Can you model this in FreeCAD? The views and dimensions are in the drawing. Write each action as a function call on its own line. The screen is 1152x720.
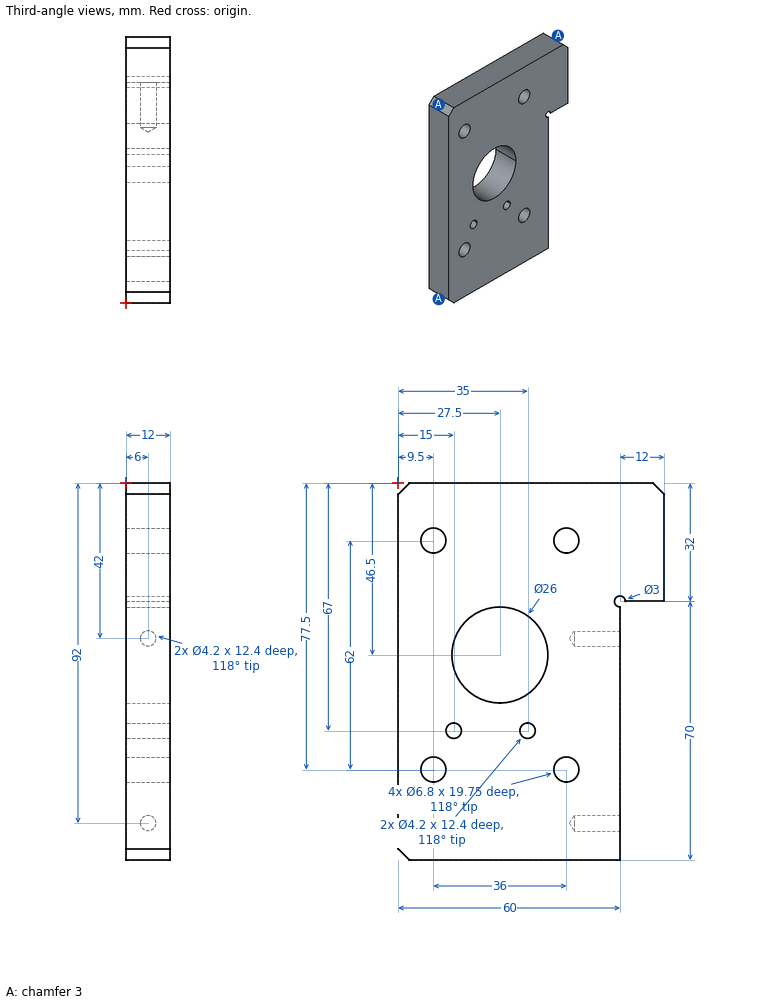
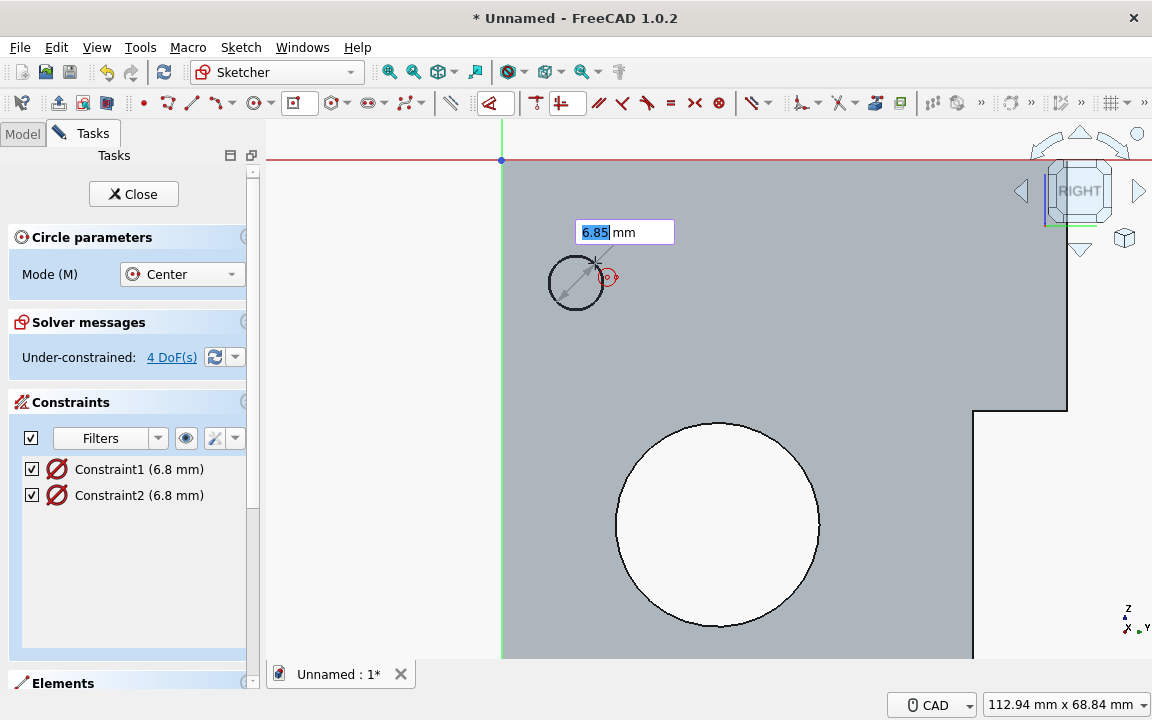
text(6.8)
key(Return)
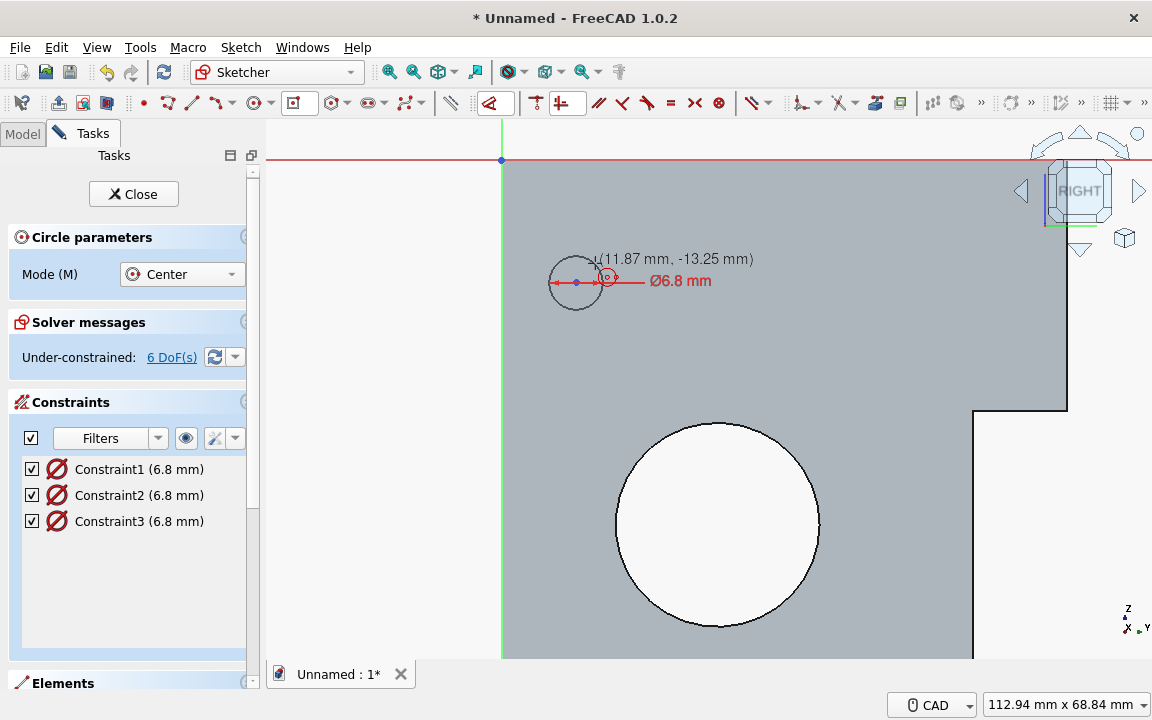
click(859, 282)
move(878, 263)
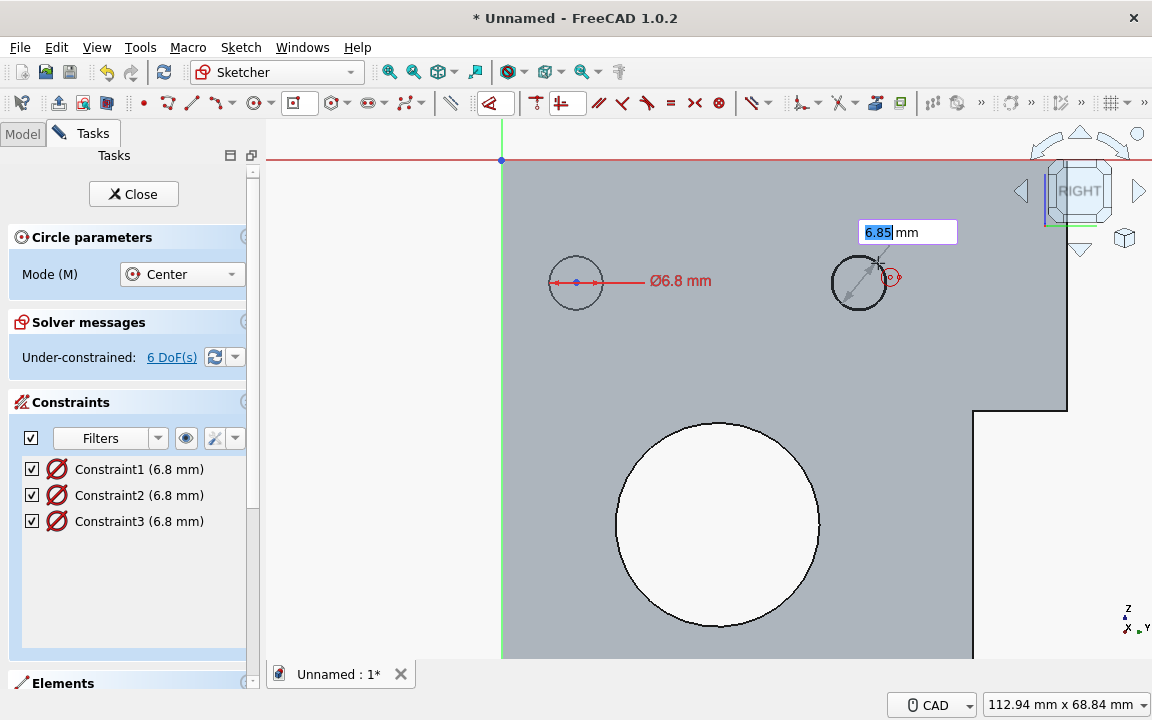
text(6.8)
key(Return)
key(Escape)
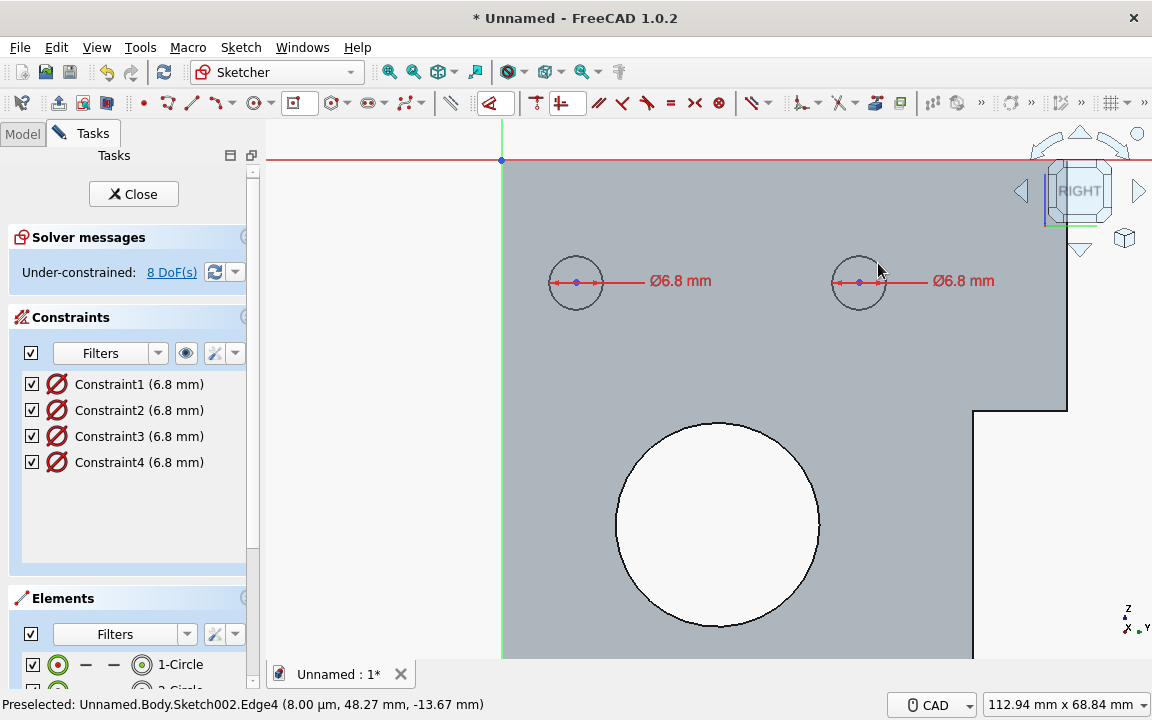
scroll(576, 281, down, 3)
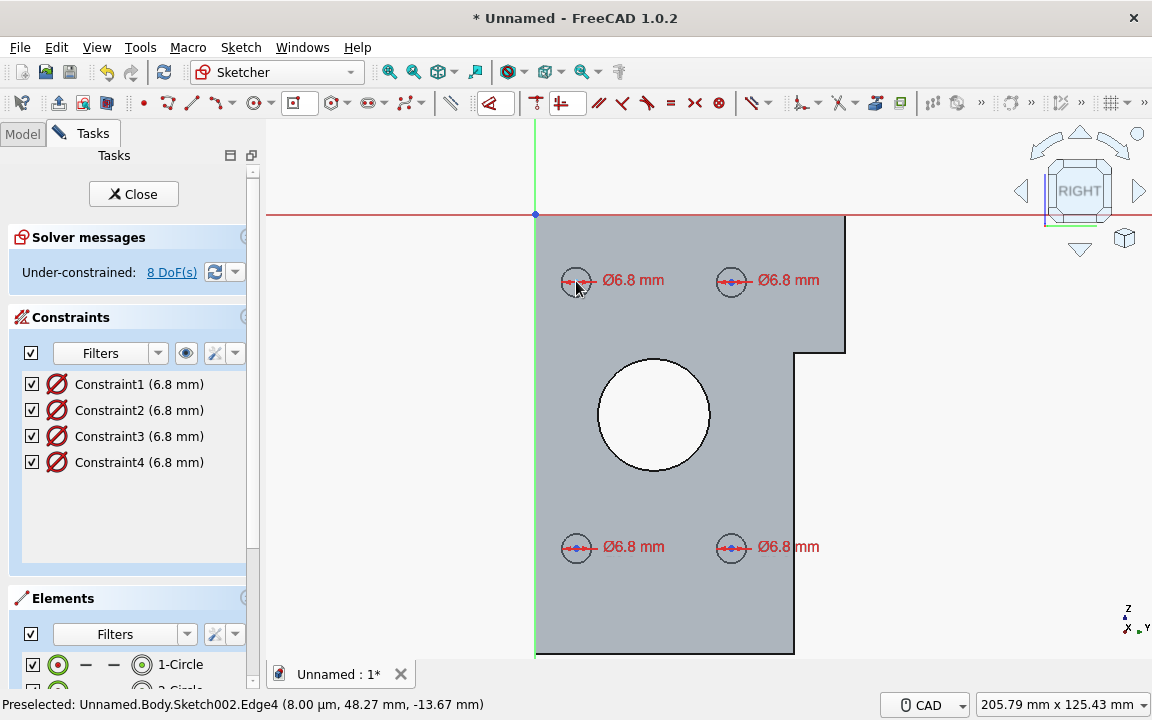
click(731, 549)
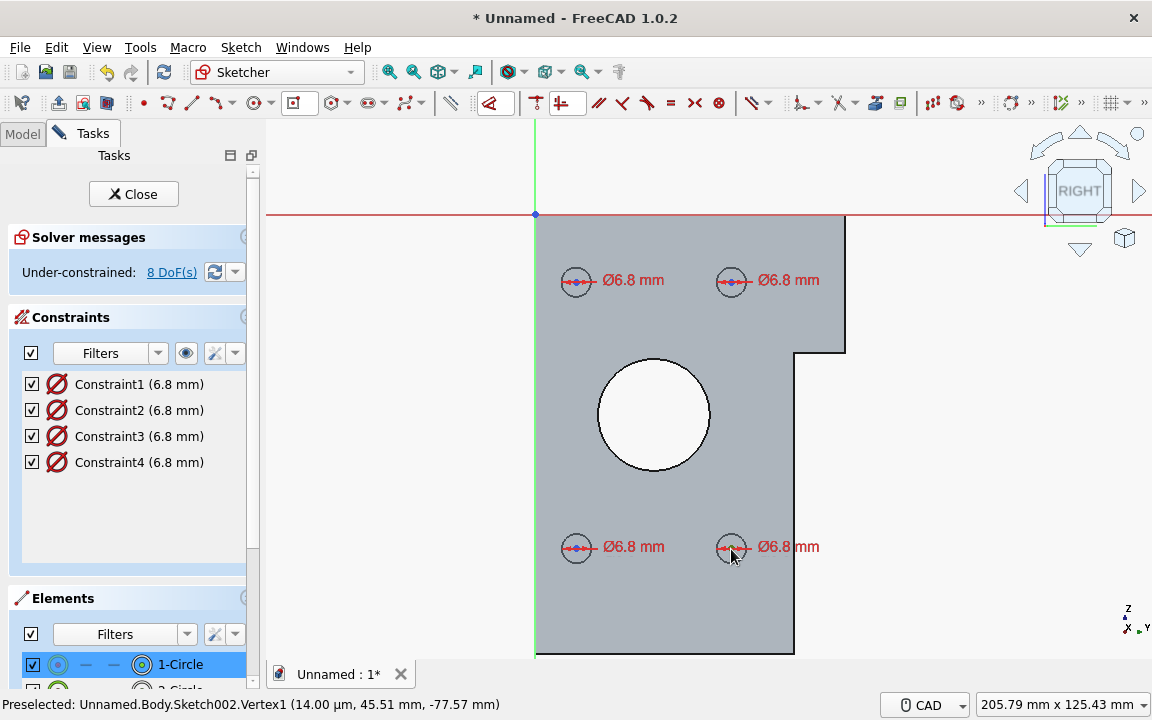
click(577, 549)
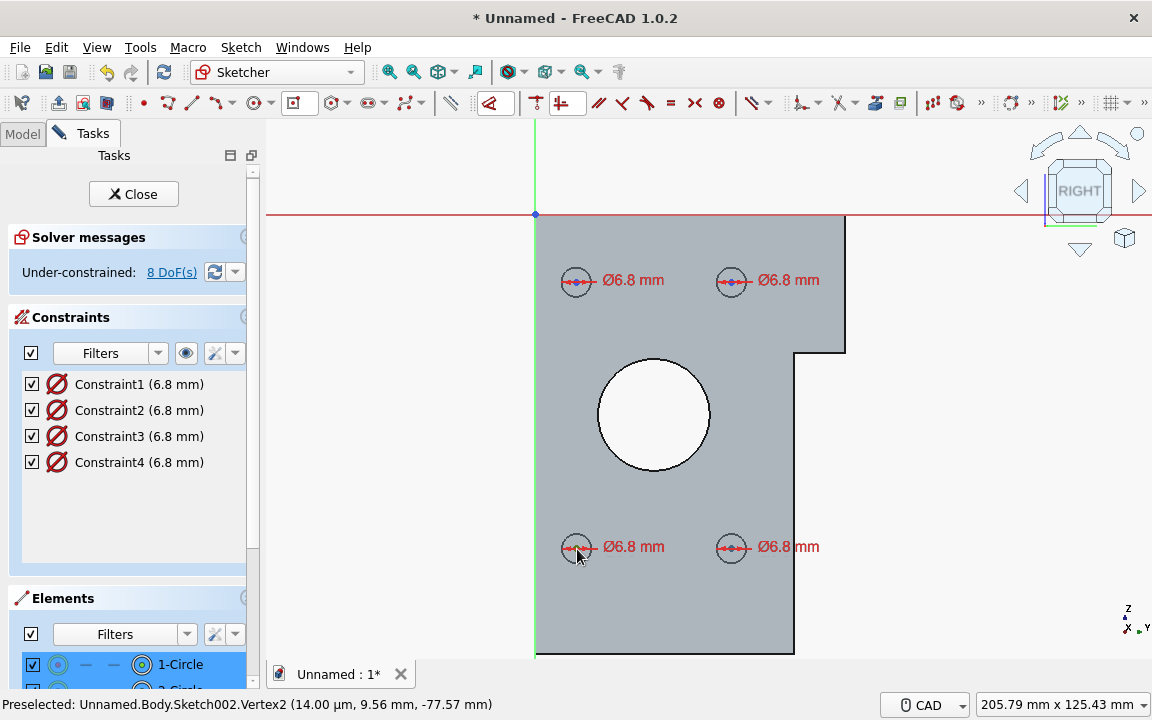
key(h)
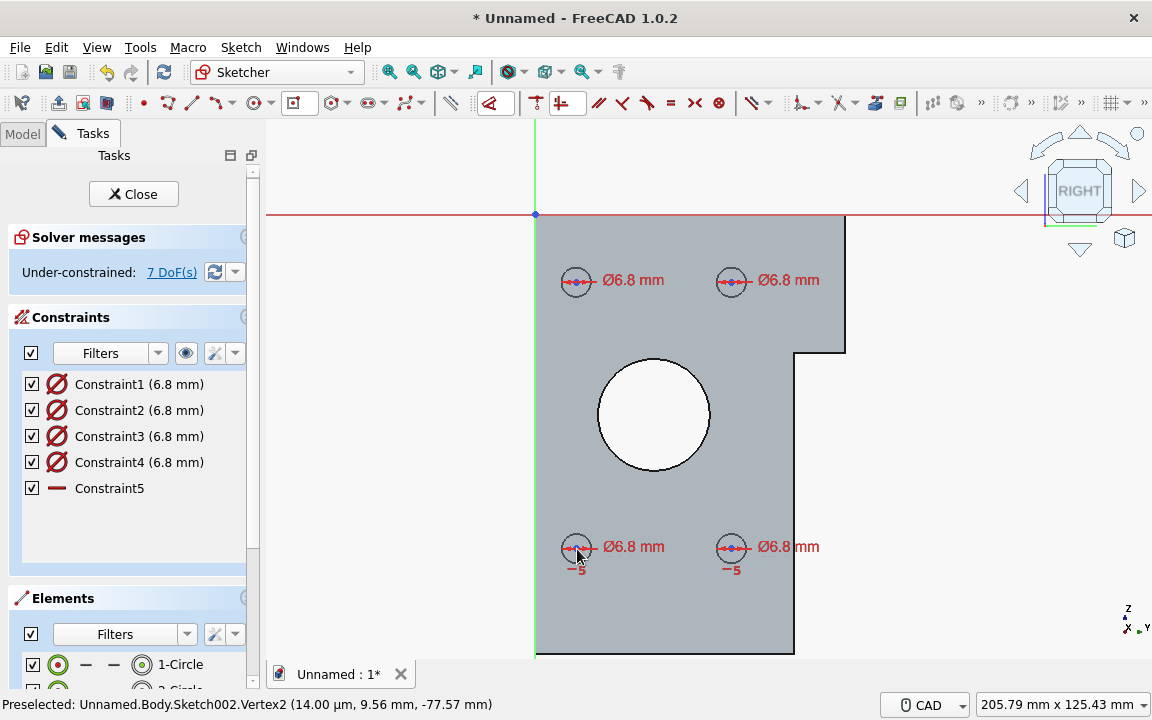
click(577, 549)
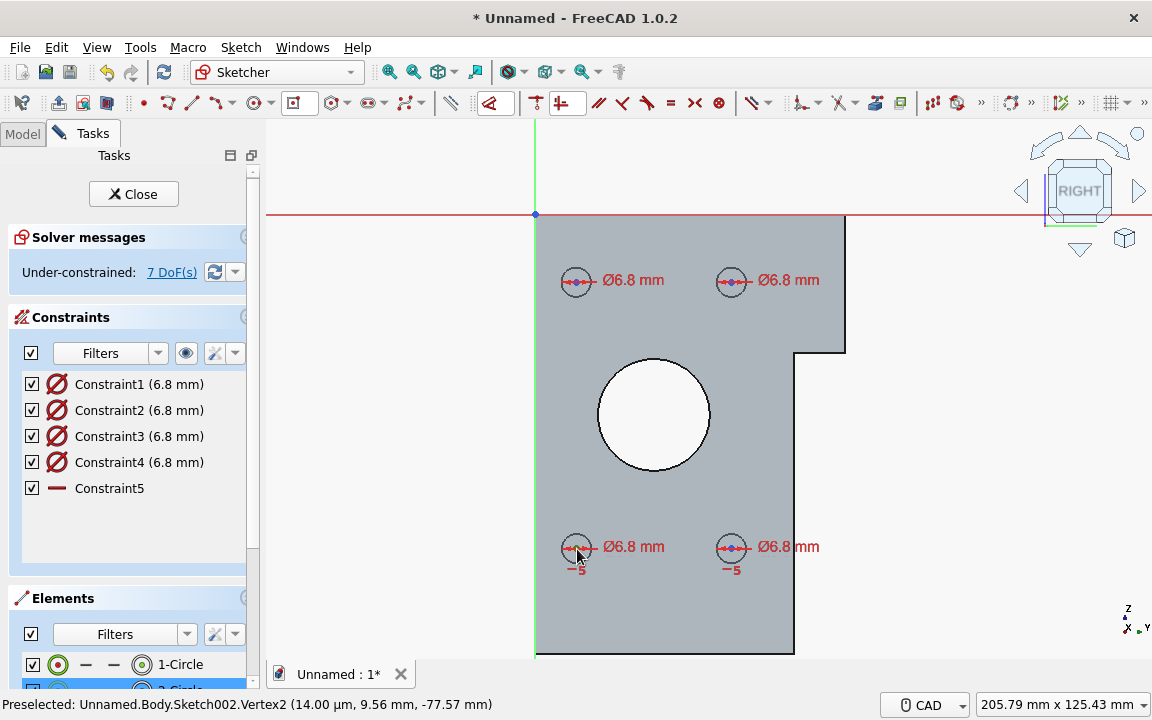
click(576, 282)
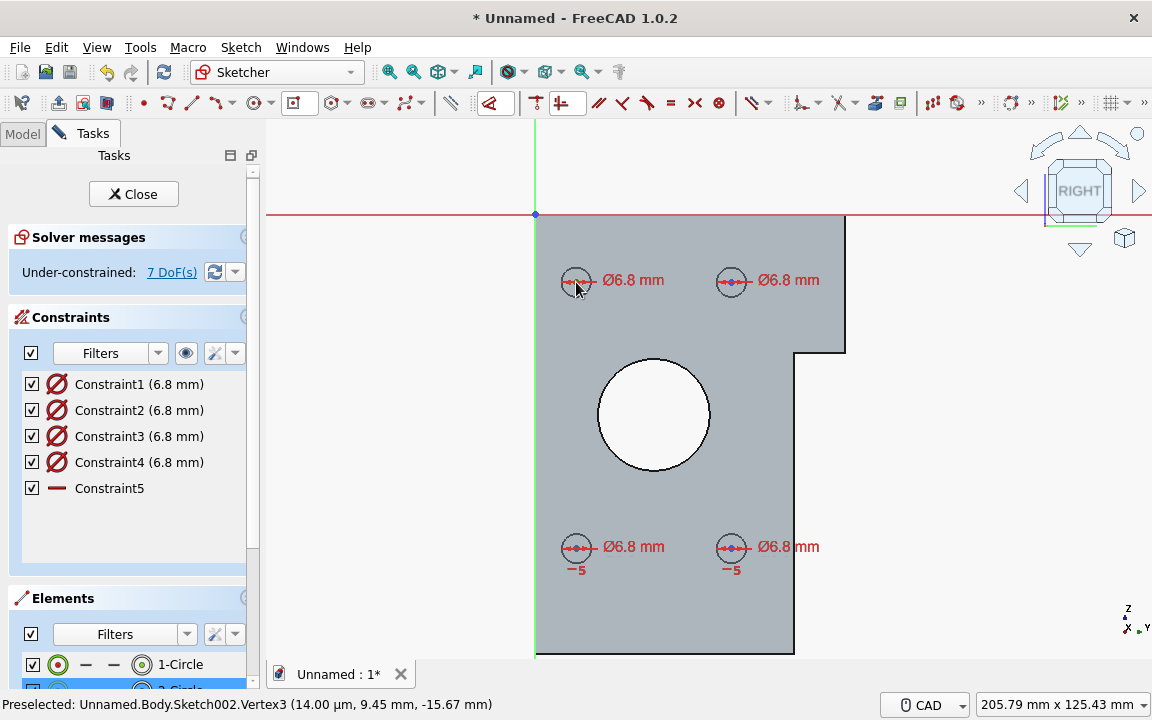
key(v)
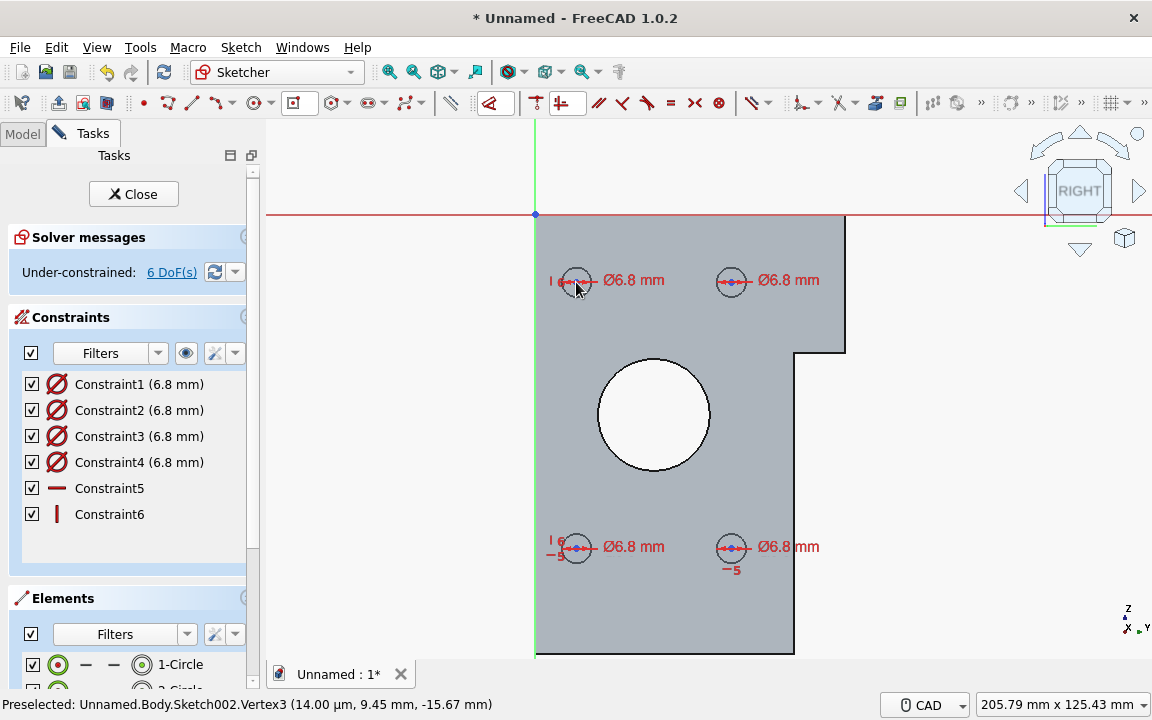
click(731, 549)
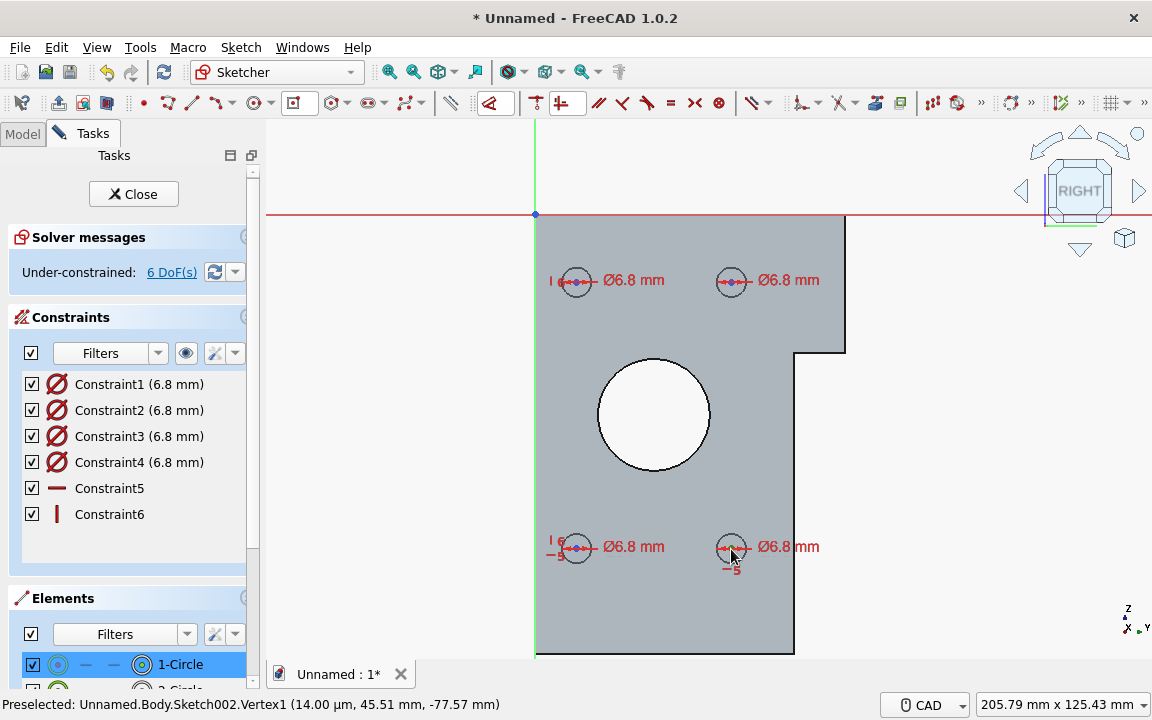
click(731, 282)